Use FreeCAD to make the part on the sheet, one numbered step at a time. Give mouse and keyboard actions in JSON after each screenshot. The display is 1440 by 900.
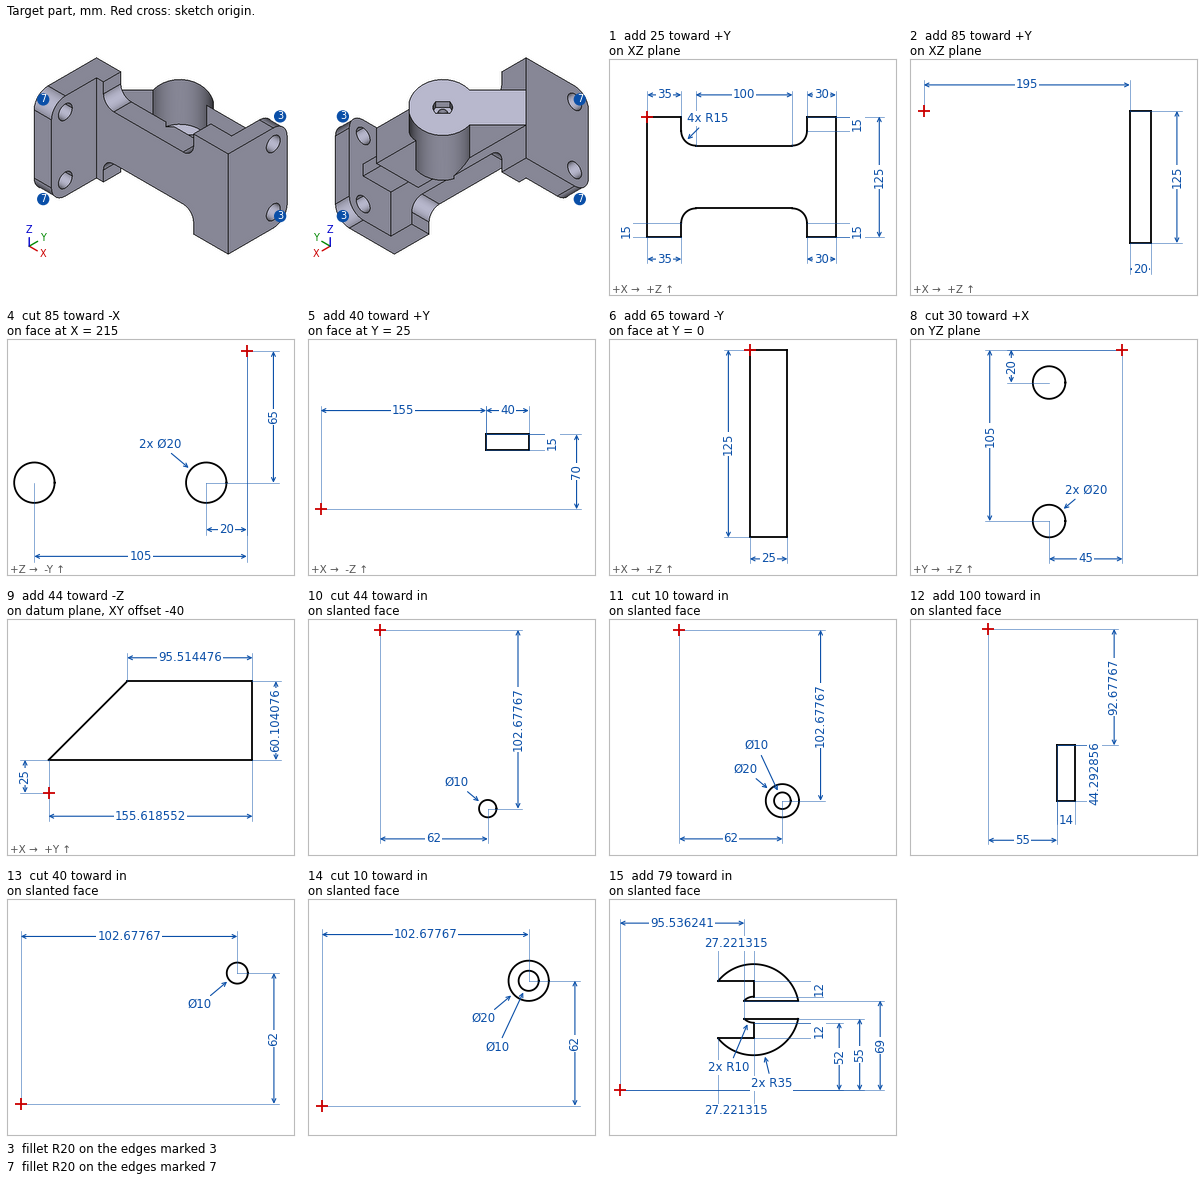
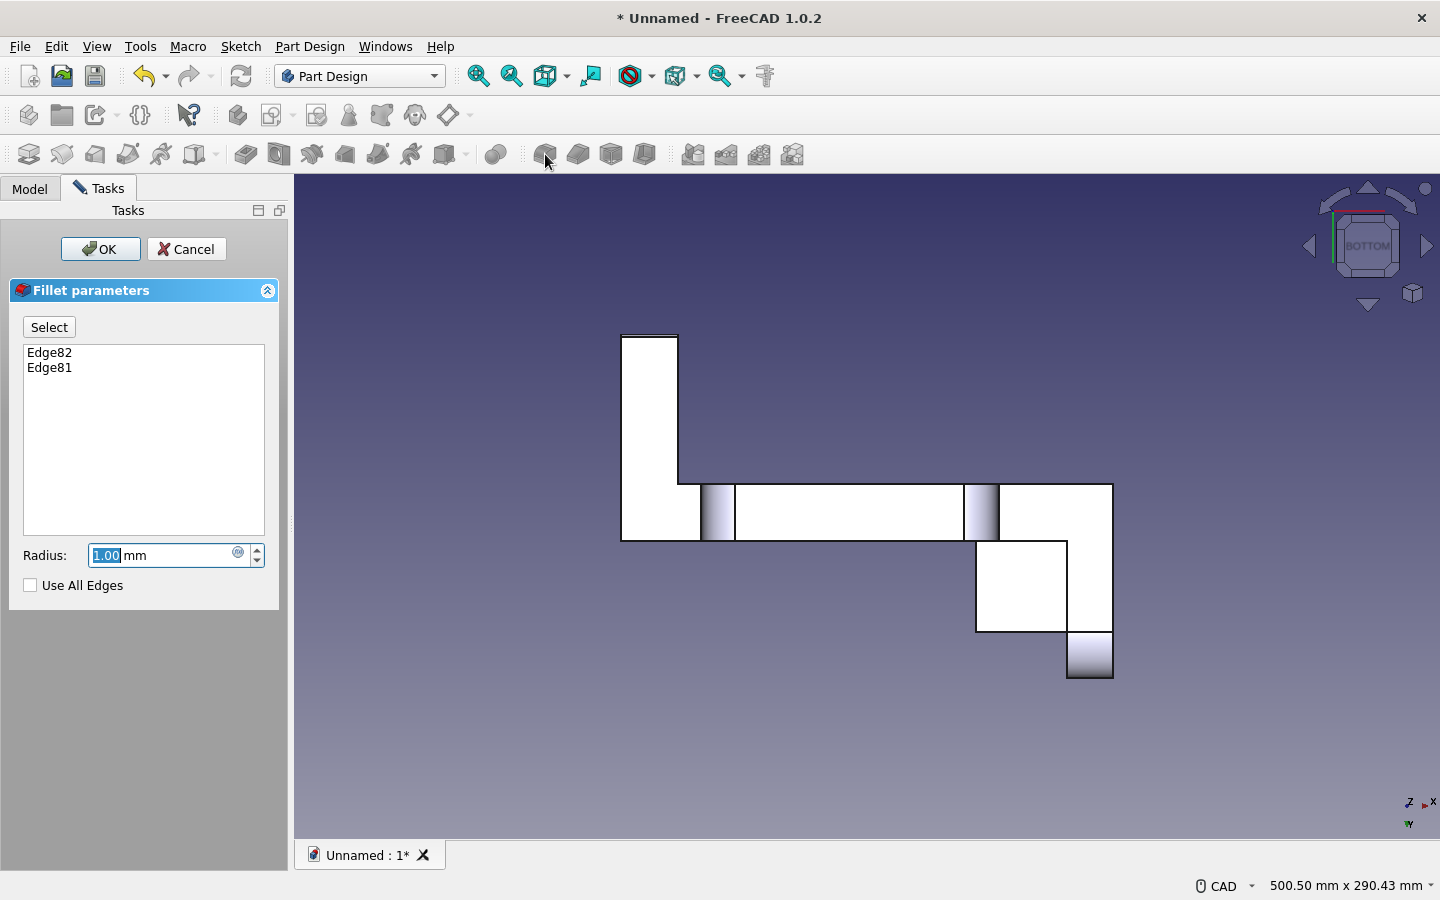
{"action": "type", "text": "20"}
{"action": "key", "text": "Tab"}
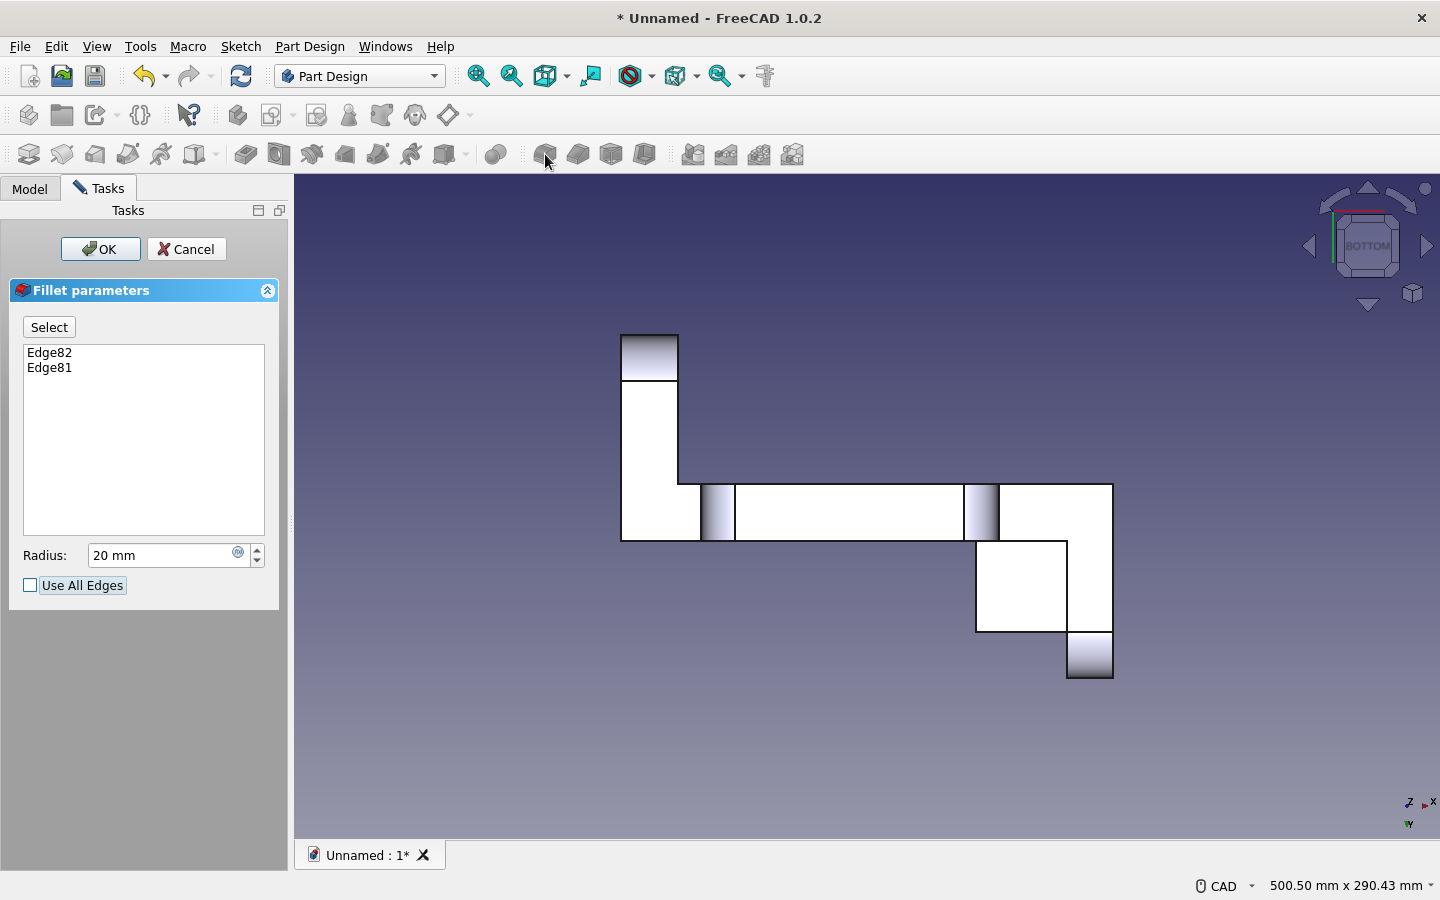
{"action": "left_click", "coordinate": [101, 249]}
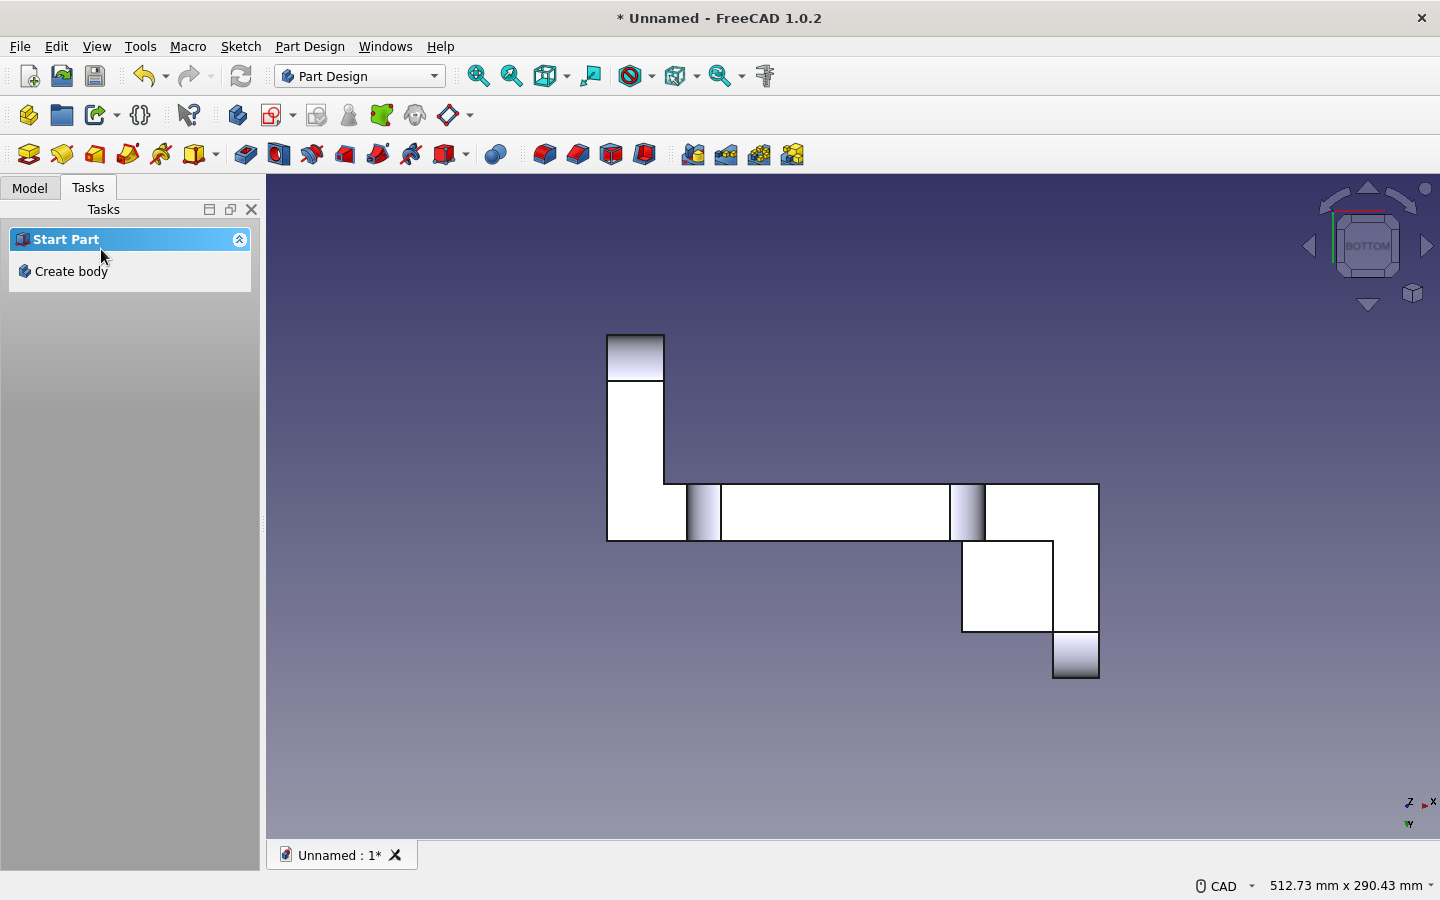
{"action": "left_click", "coordinate": [270, 116]}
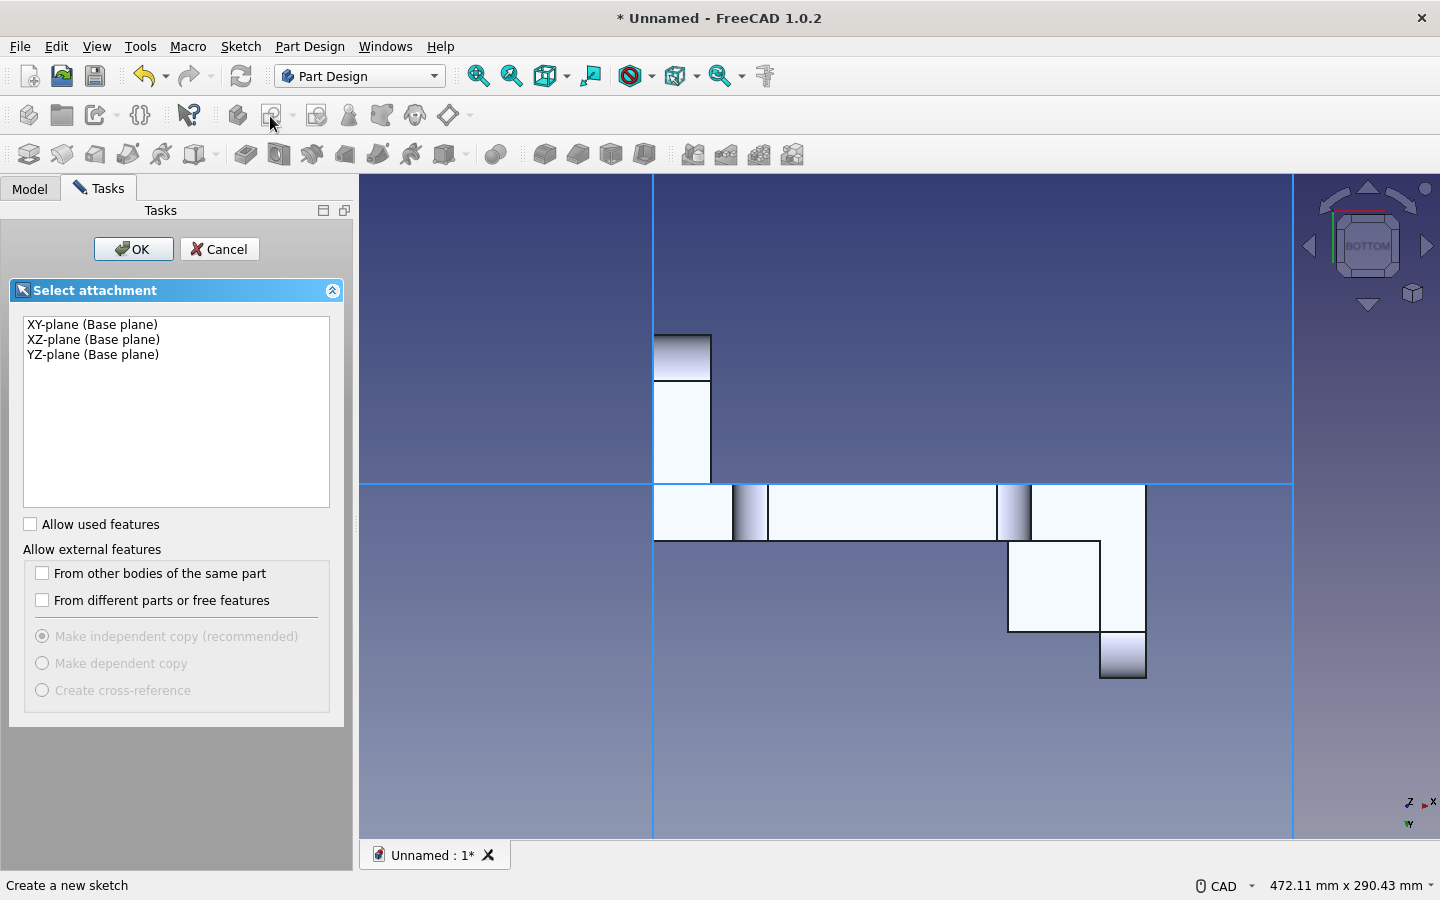
{"action": "left_click", "coordinate": [84, 354]}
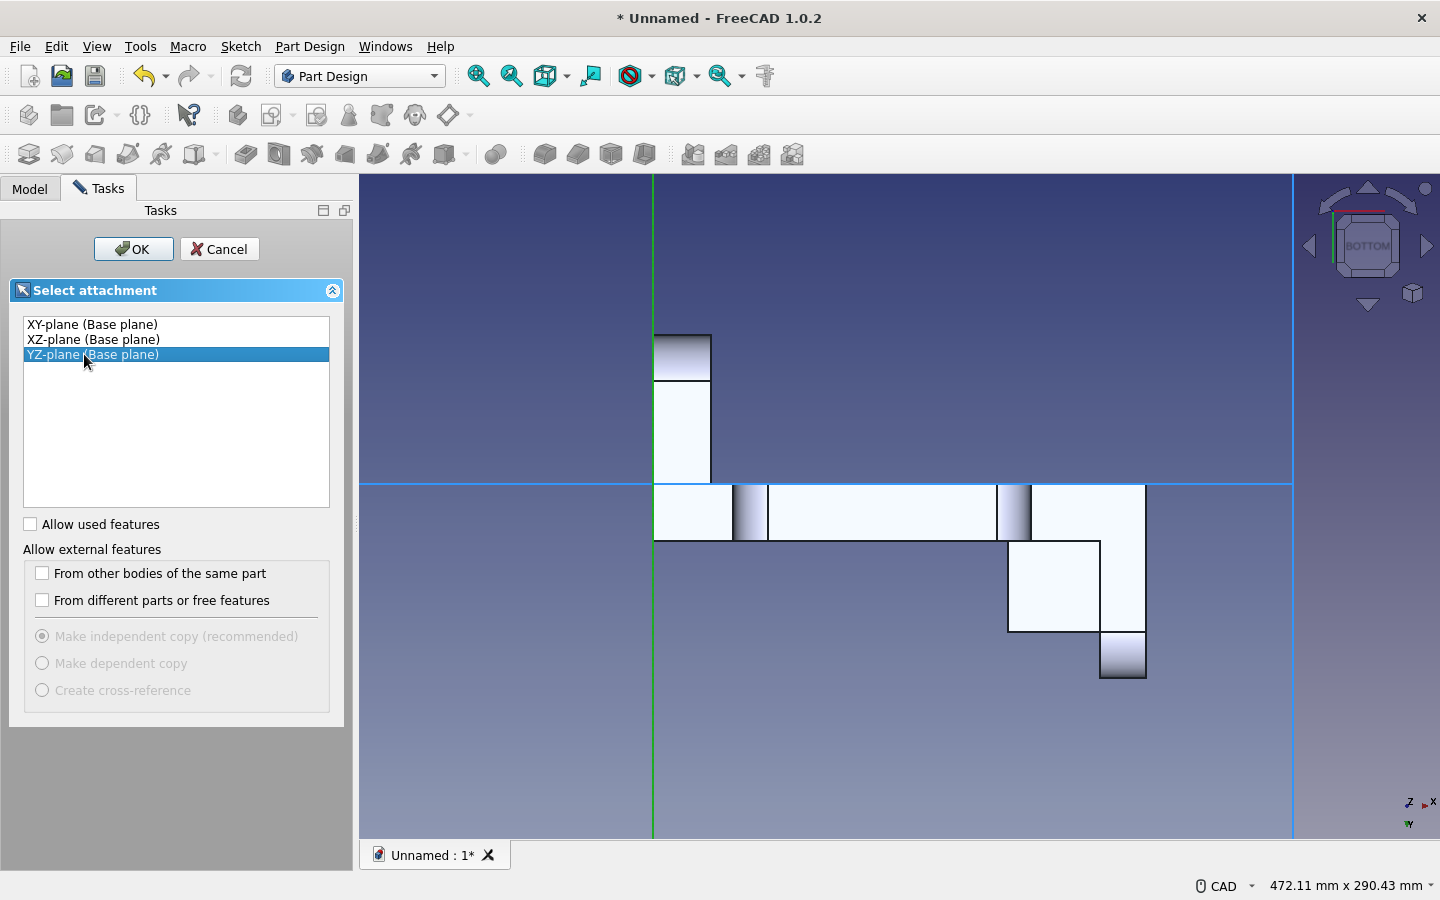
{"action": "left_click", "coordinate": [134, 249]}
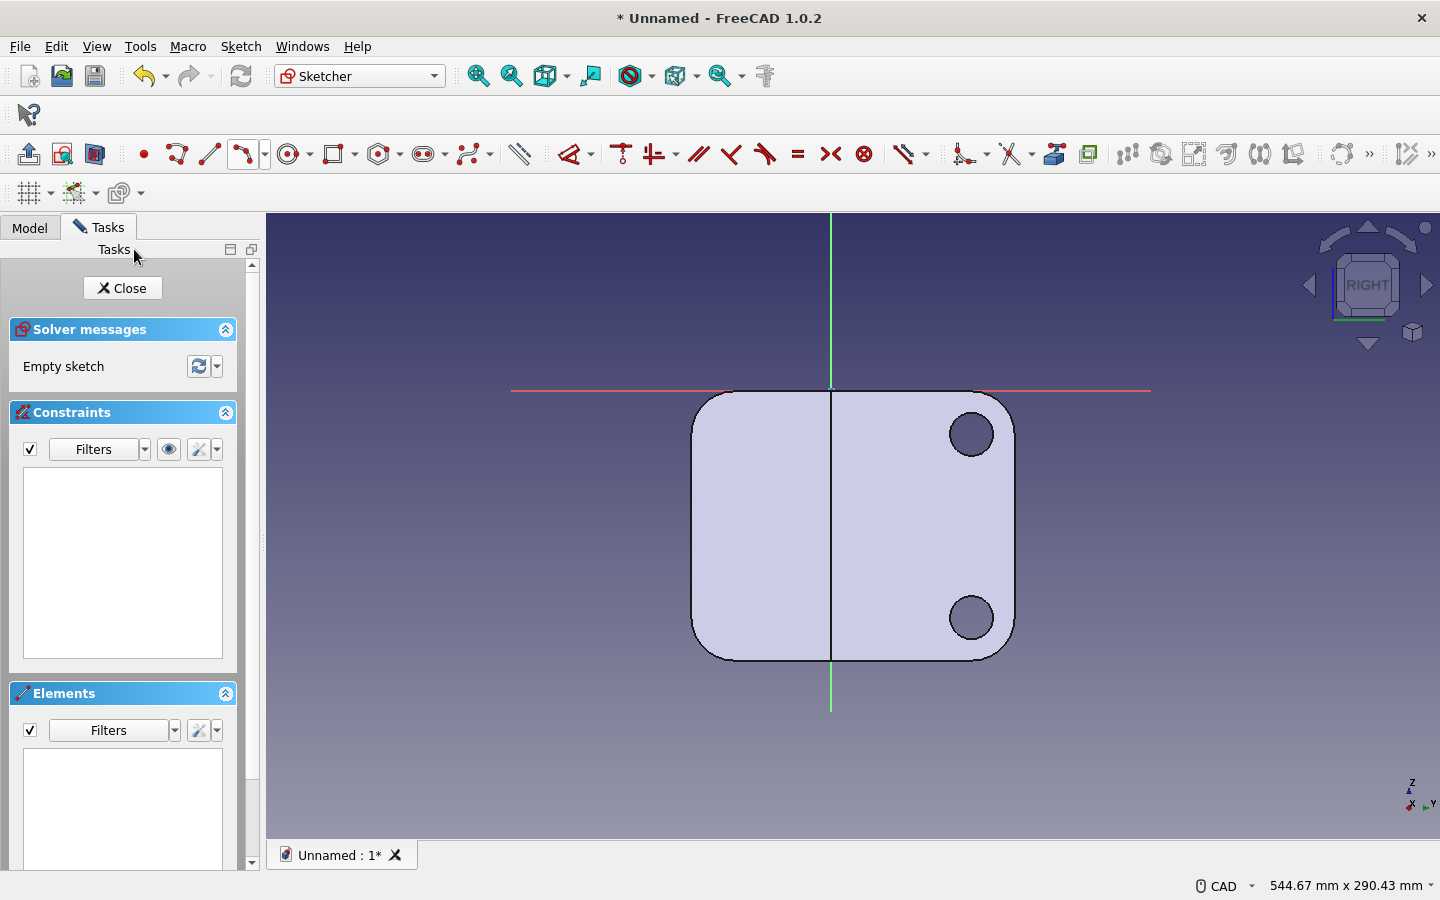
{"action": "left_click", "coordinate": [95, 154]}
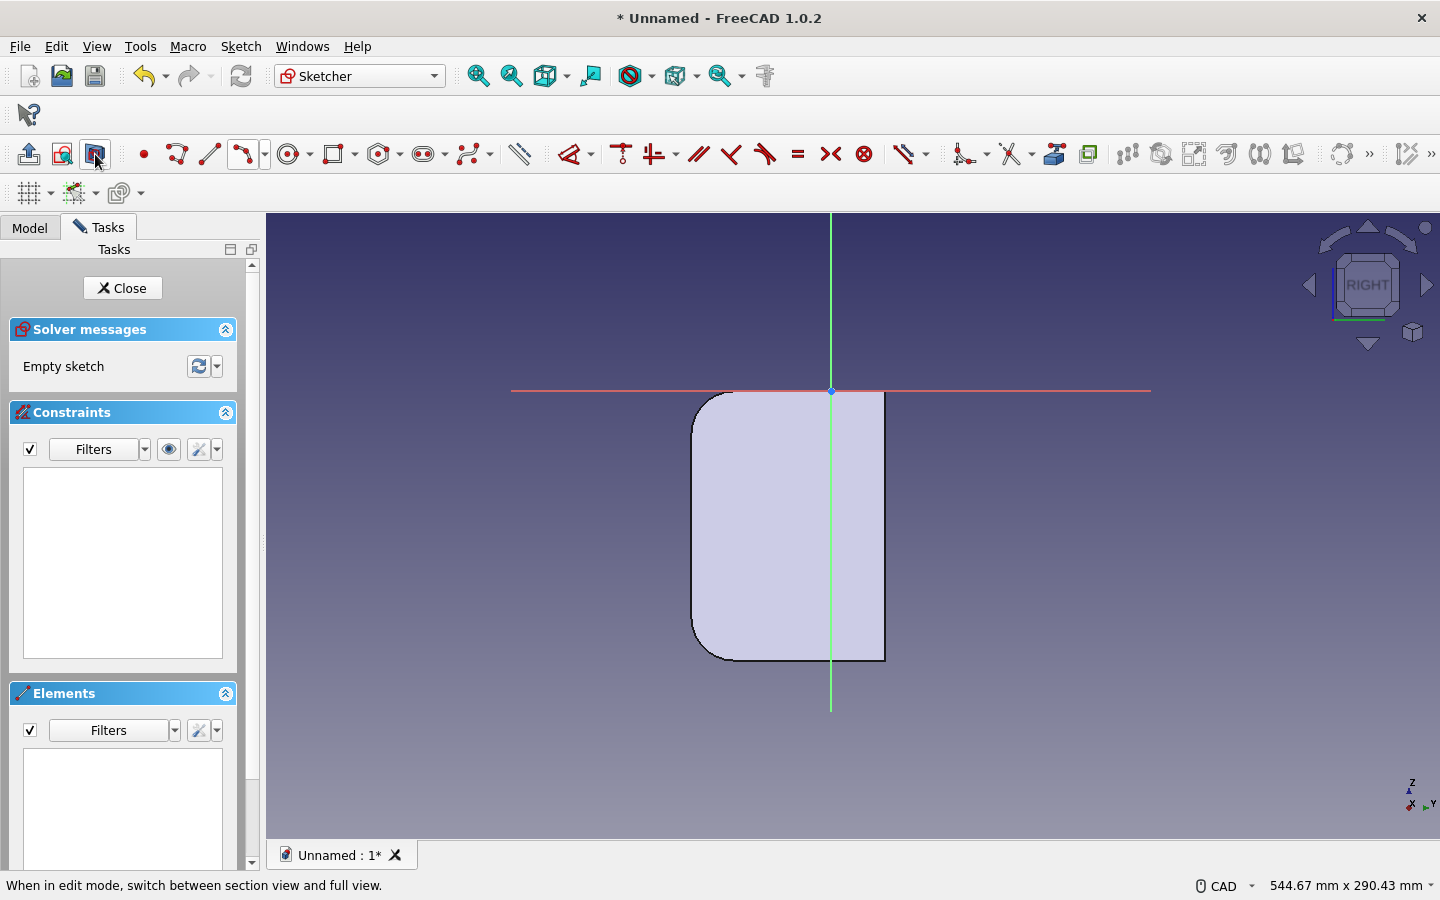
{"action": "scroll", "coordinate": [747, 493], "scroll_direction": "up", "scroll_amount": 2}